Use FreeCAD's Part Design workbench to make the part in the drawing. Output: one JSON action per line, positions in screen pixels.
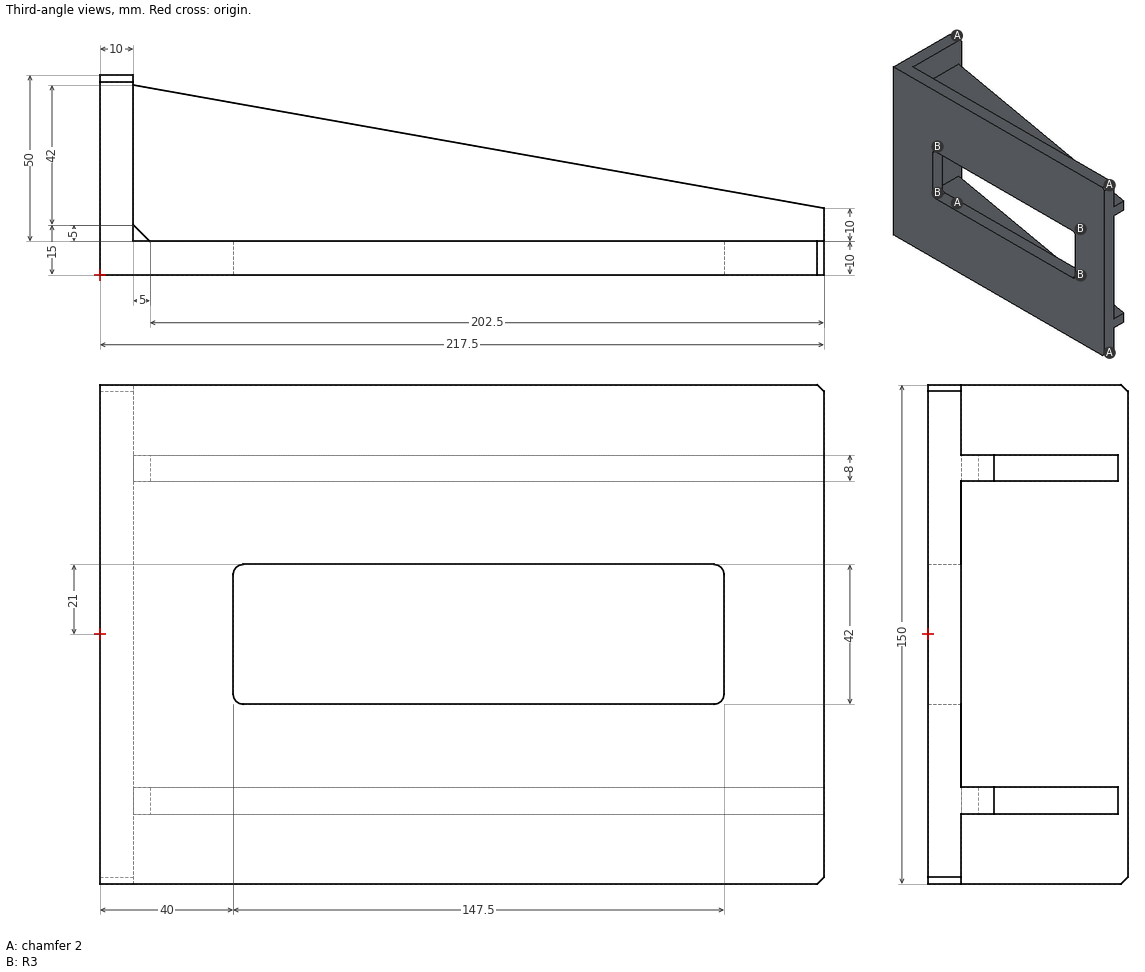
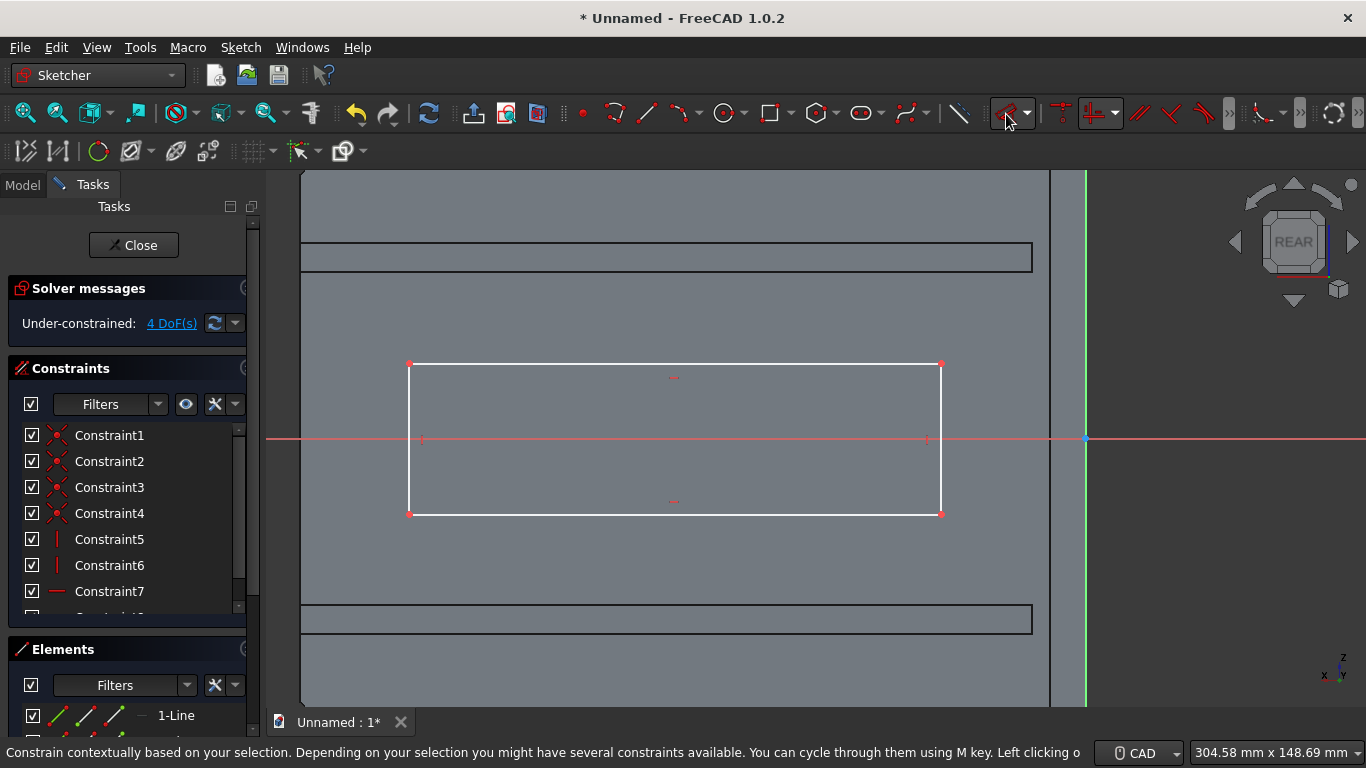
{"action": "left_click", "coordinate": [409, 409]}
{"action": "left_click", "coordinate": [375, 405]}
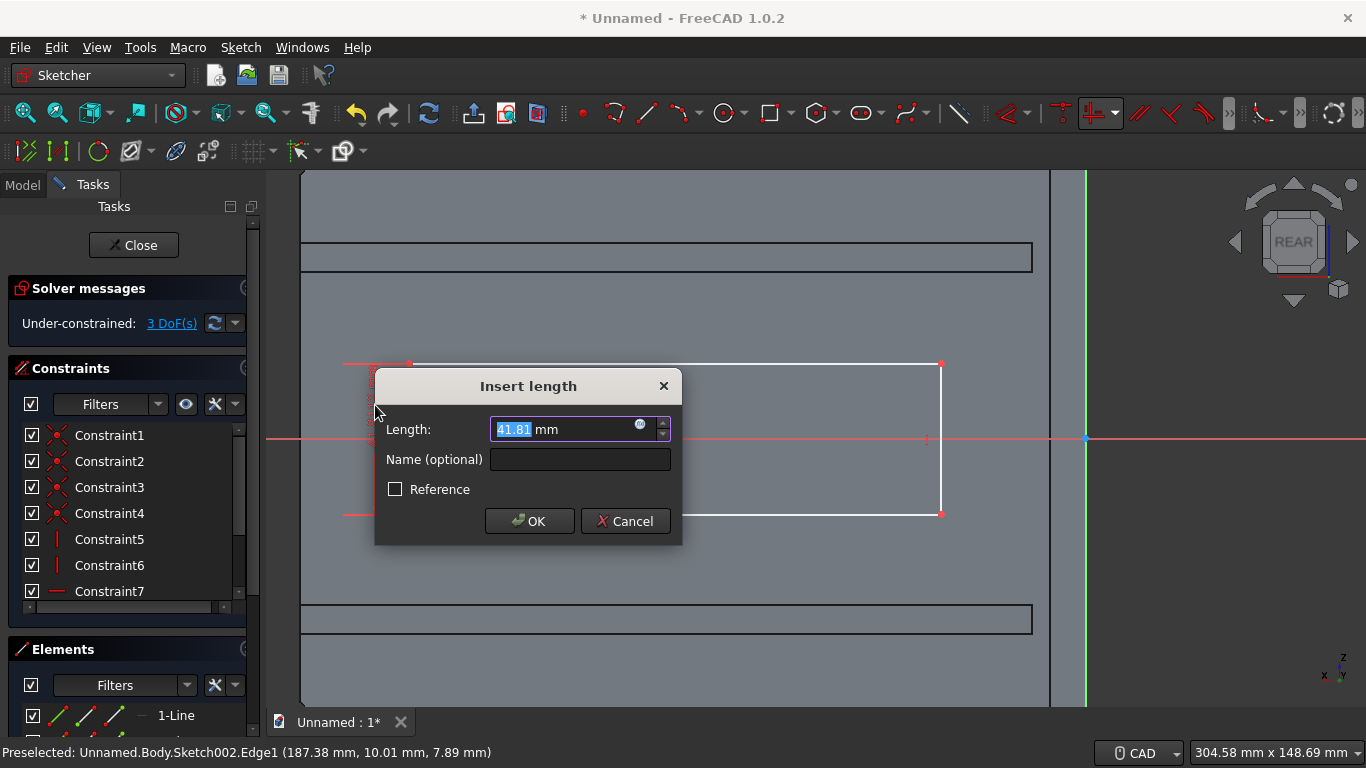
{"action": "type", "text": "42"}
{"action": "key", "text": "Return"}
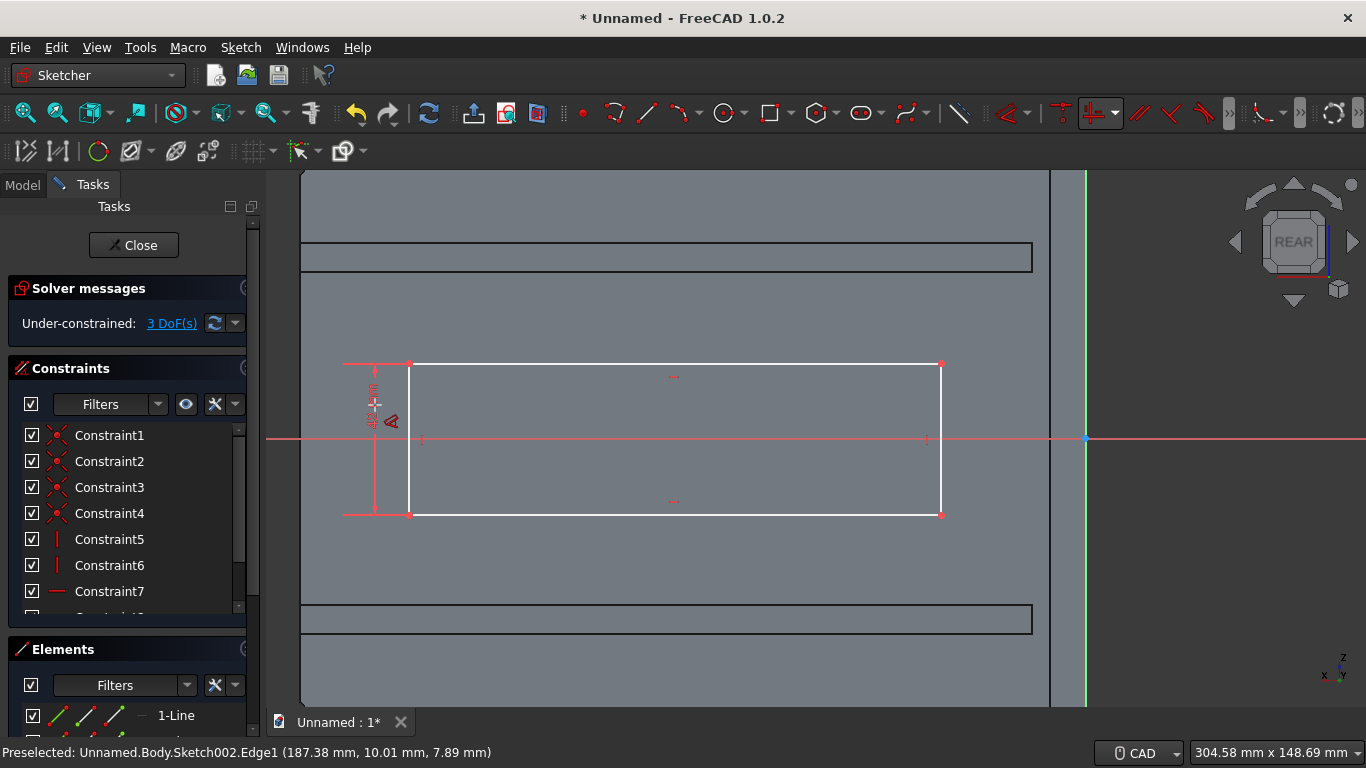
{"action": "left_click", "coordinate": [409, 364]}
{"action": "left_click", "coordinate": [1120, 401]}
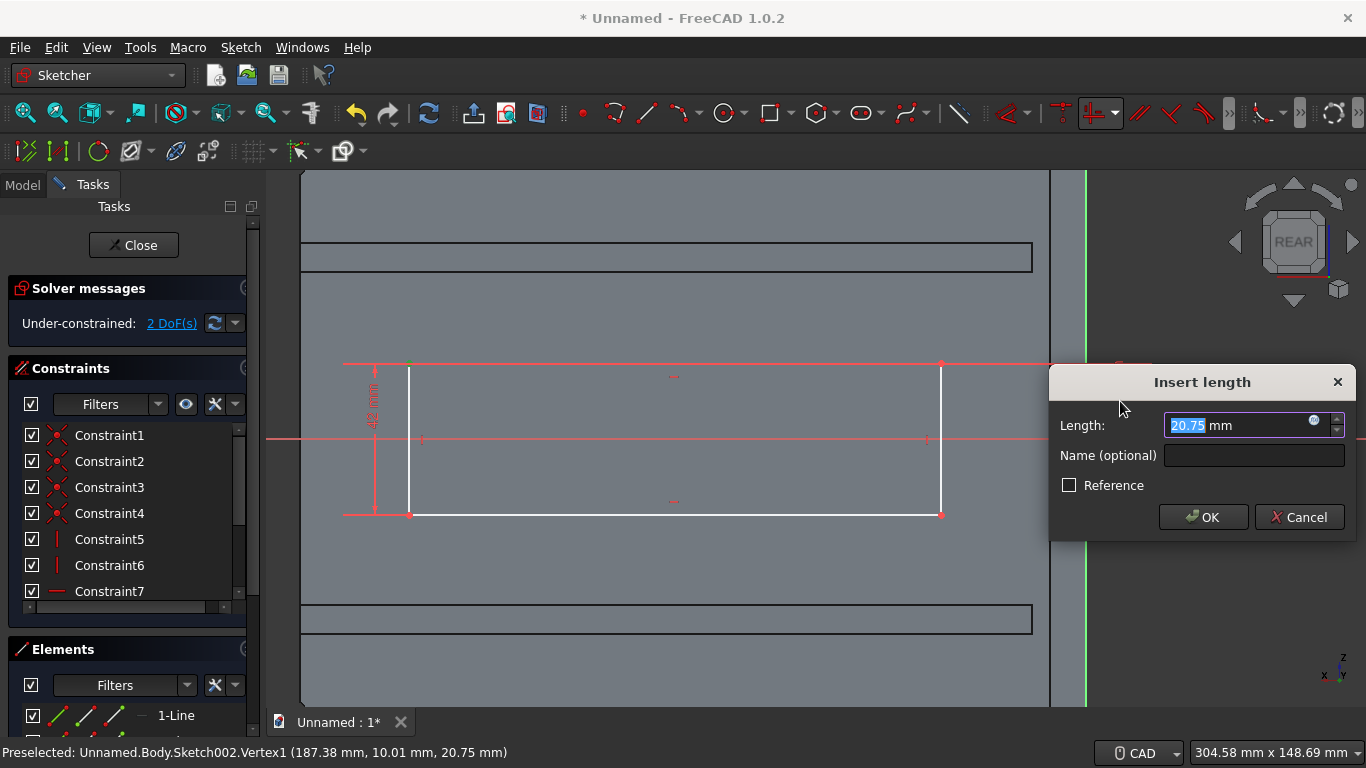
{"action": "type", "text": "21"}
{"action": "key", "text": "Return"}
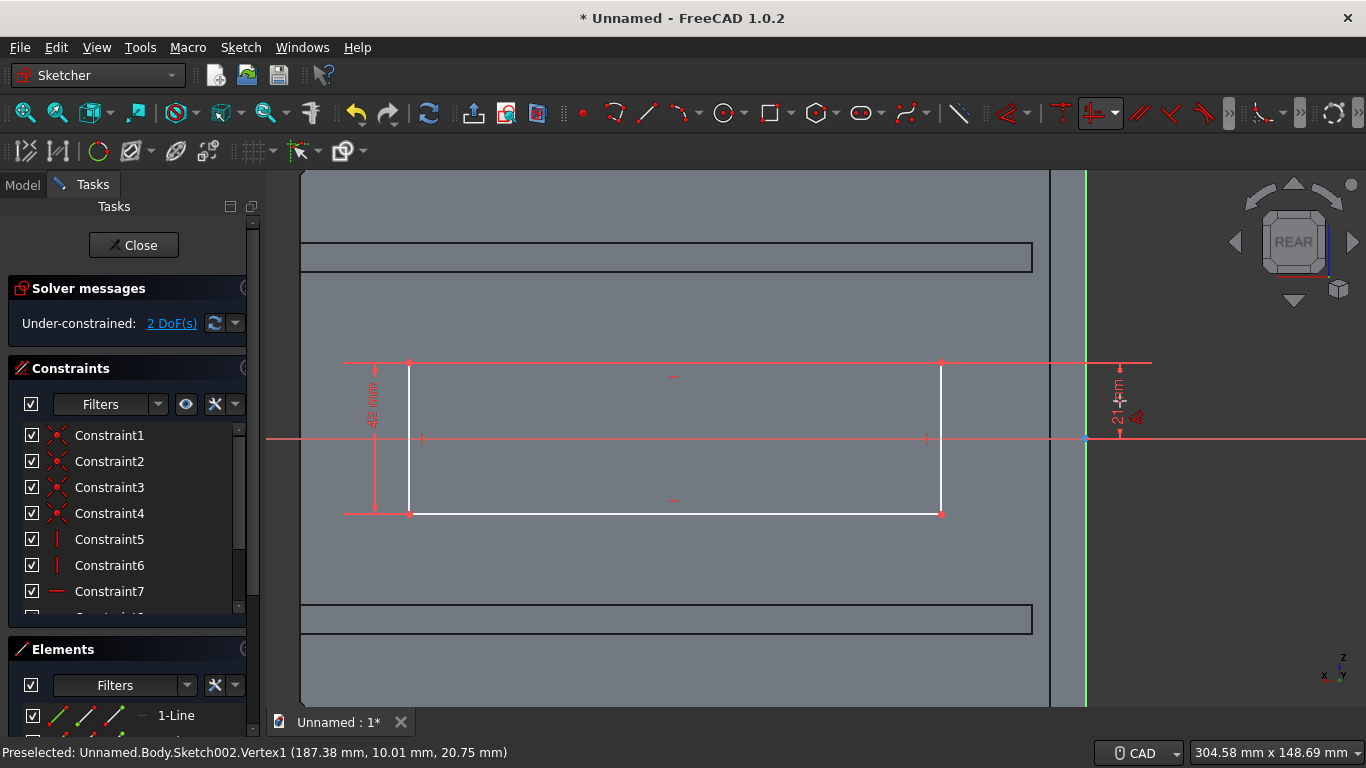
{"action": "left_click", "coordinate": [941, 514]}
{"action": "left_click", "coordinate": [1013, 548]}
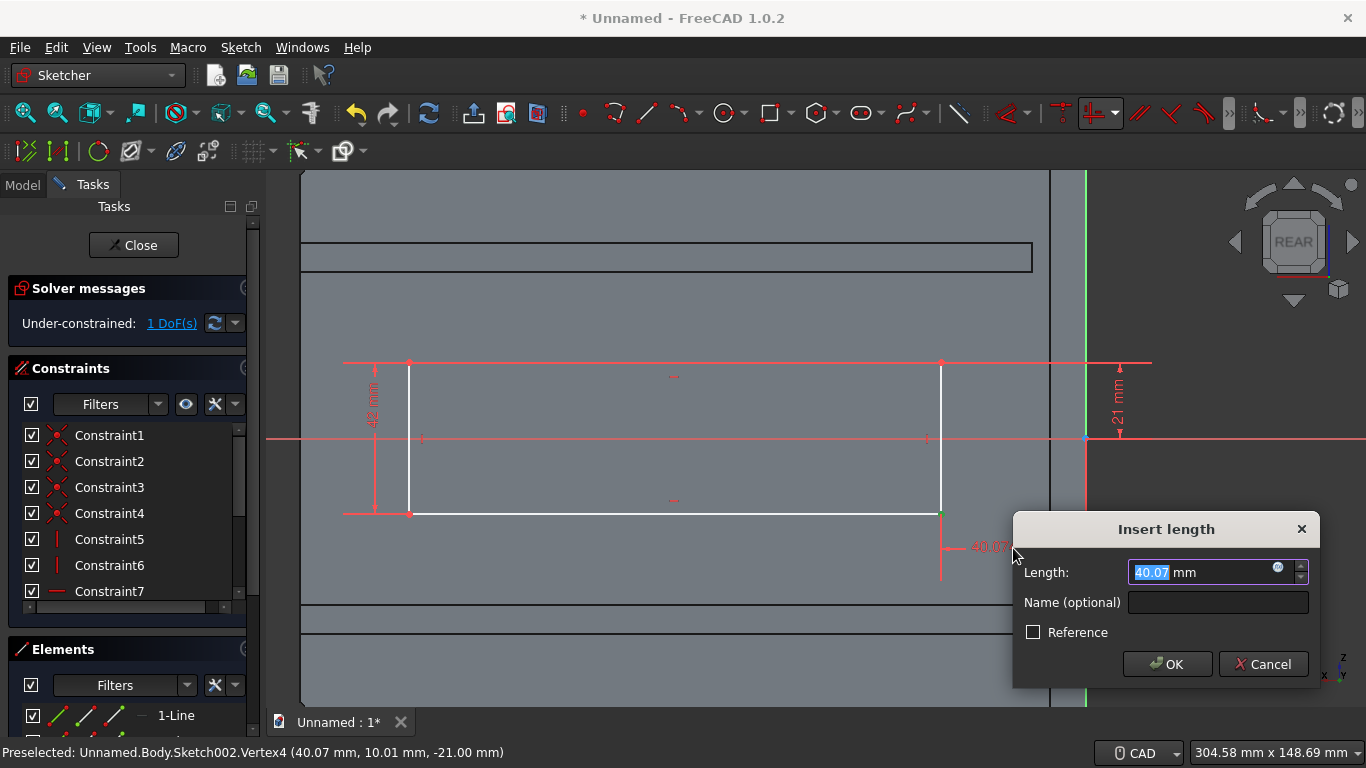
{"action": "type", "text": "40"}
{"action": "key", "text": "Return"}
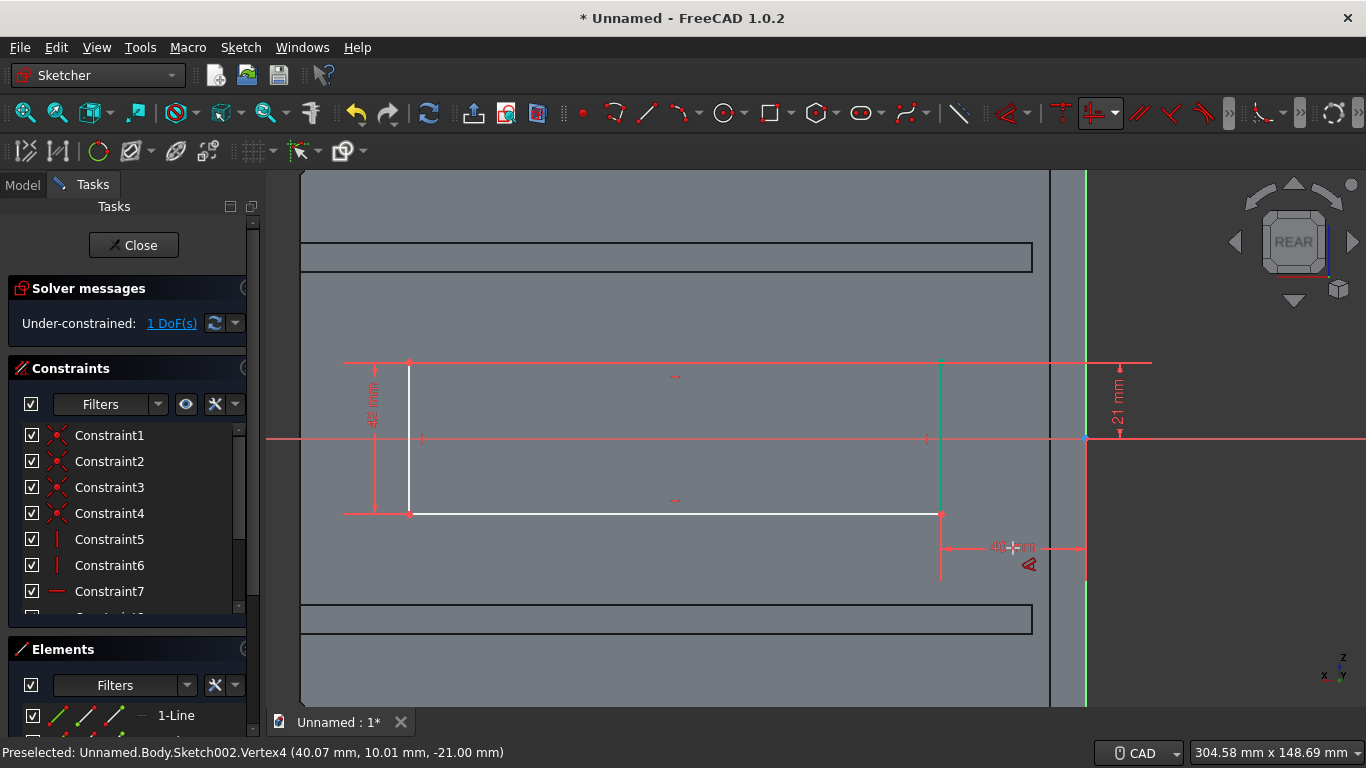
{"action": "left_click", "coordinate": [569, 514]}
{"action": "left_click", "coordinate": [675, 548]}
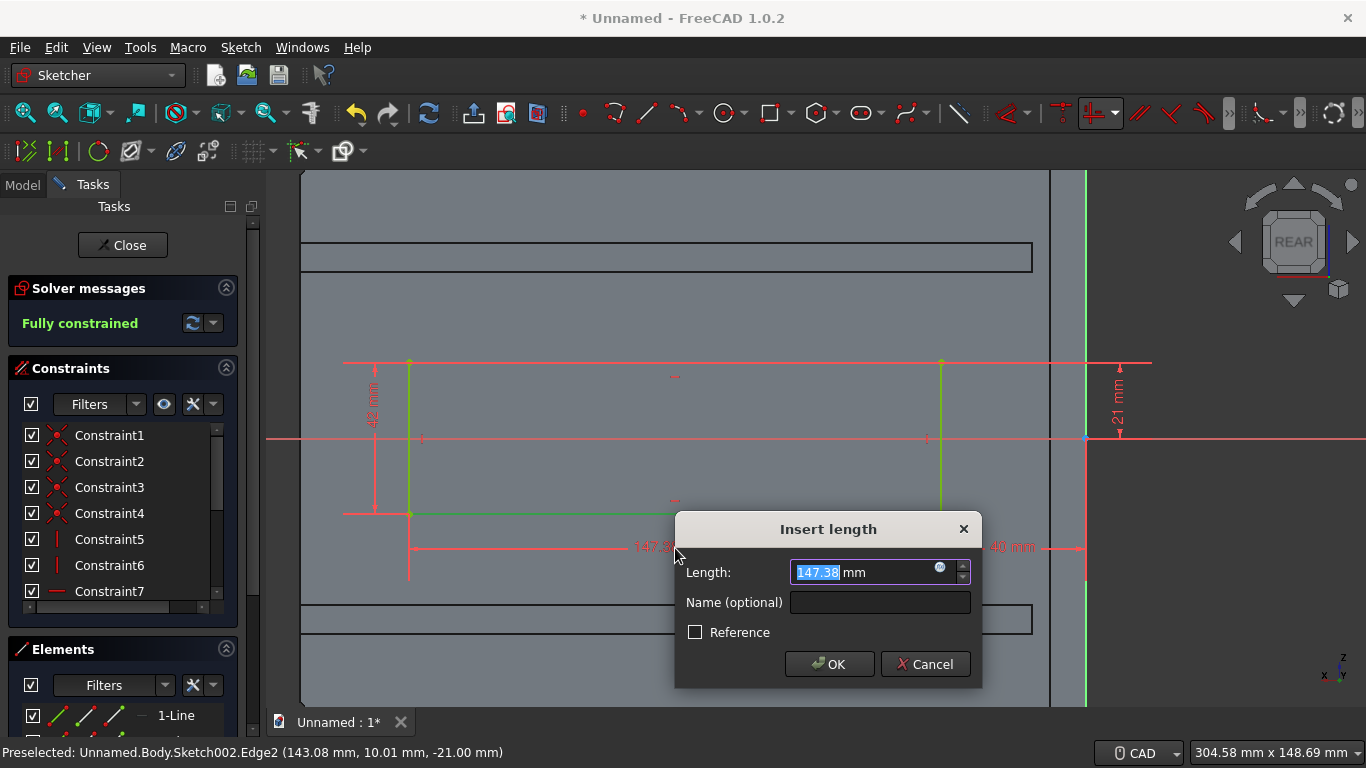
{"action": "type", "text": "147.5"}
{"action": "key", "text": "Return"}
{"action": "key", "text": "Escape"}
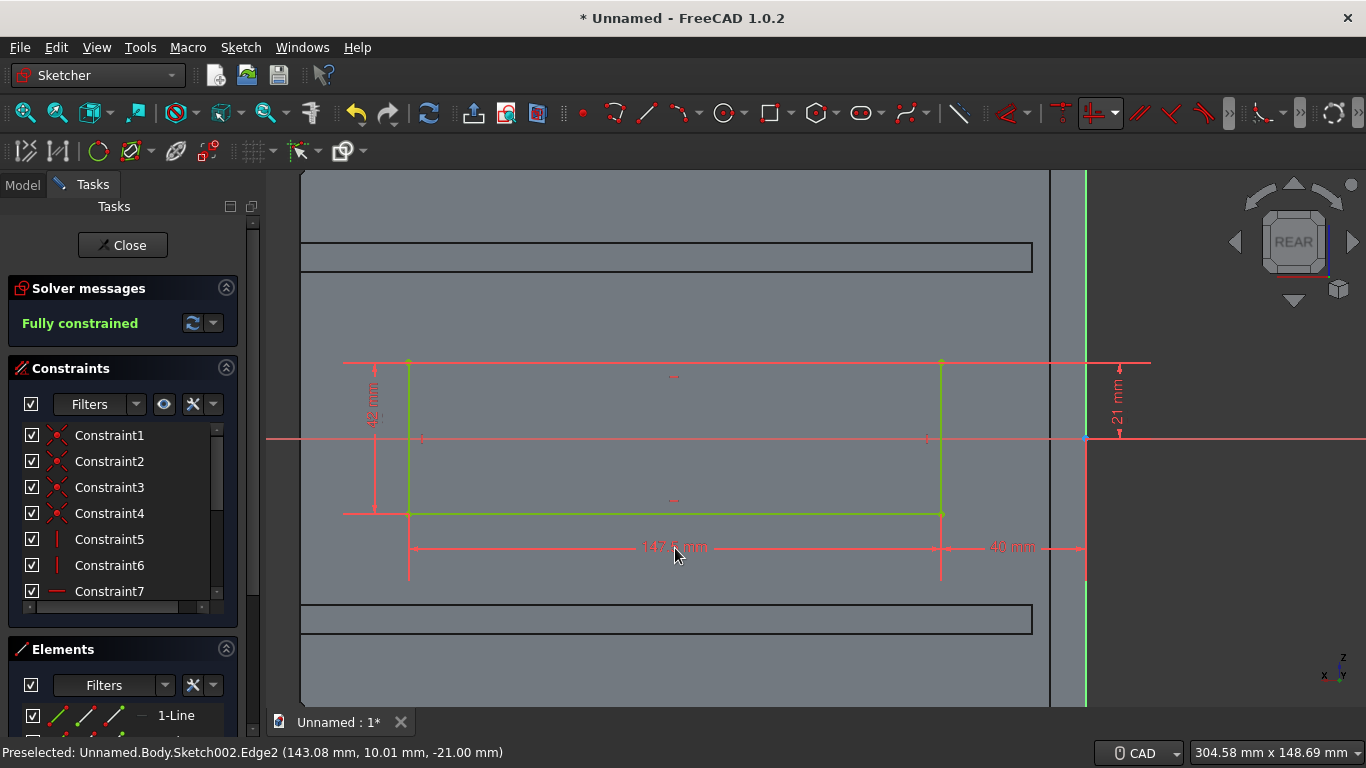
{"action": "left_click", "coordinate": [123, 245]}